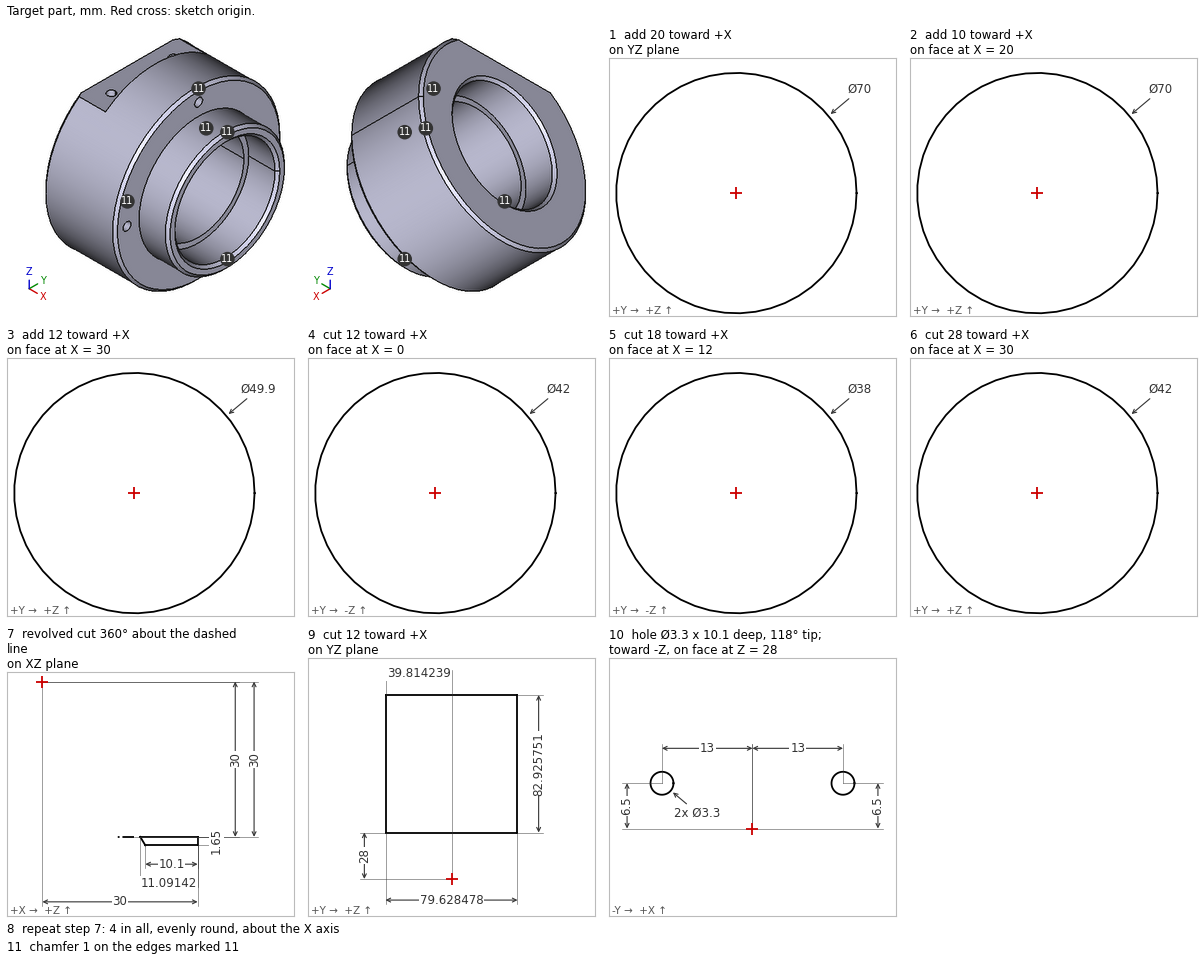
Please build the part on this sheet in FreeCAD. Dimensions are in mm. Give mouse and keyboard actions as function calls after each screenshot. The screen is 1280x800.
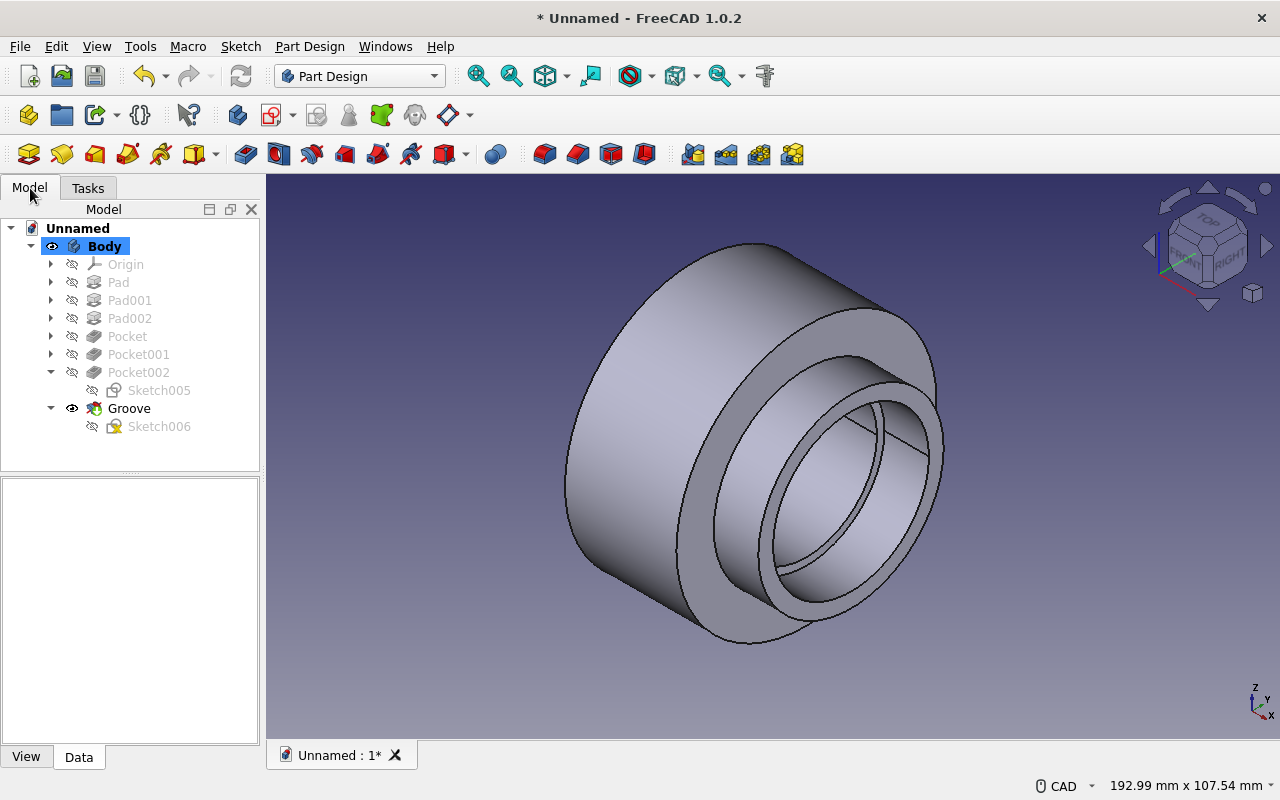
click(117, 408)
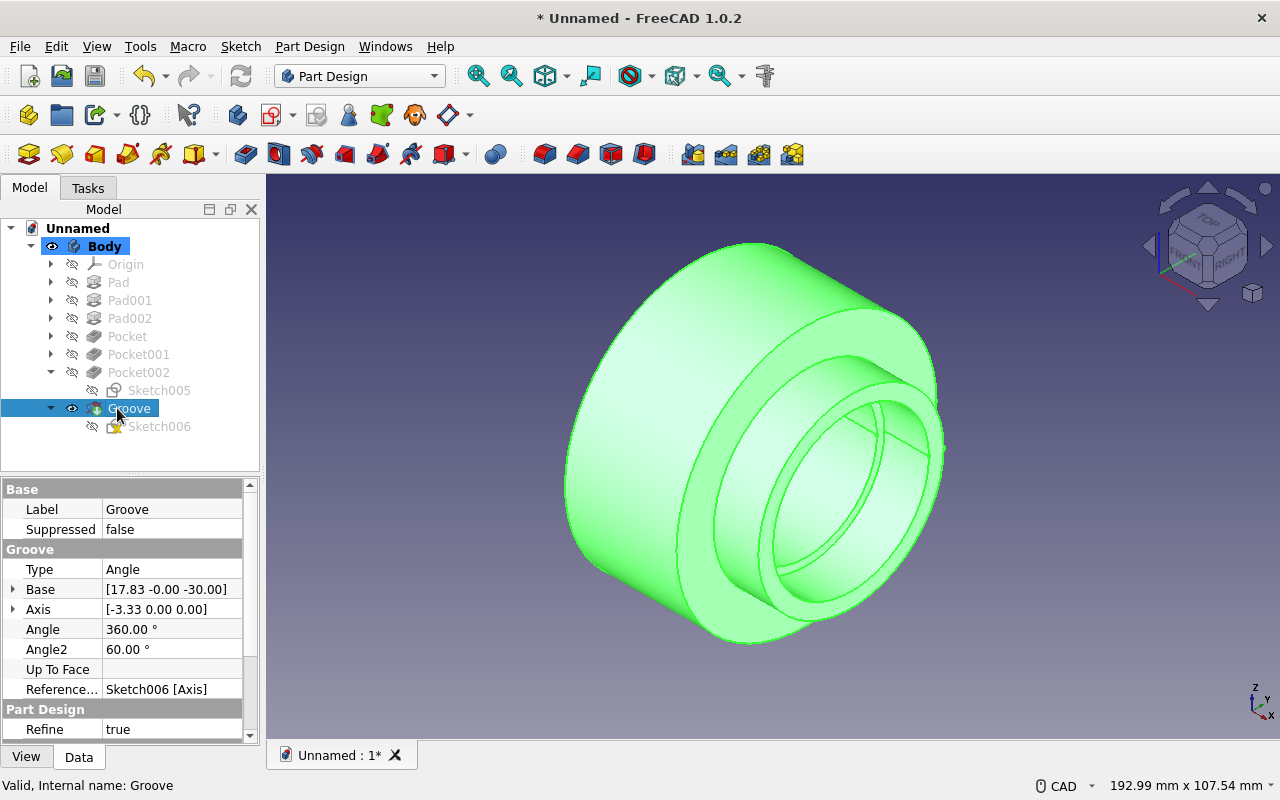
click(759, 154)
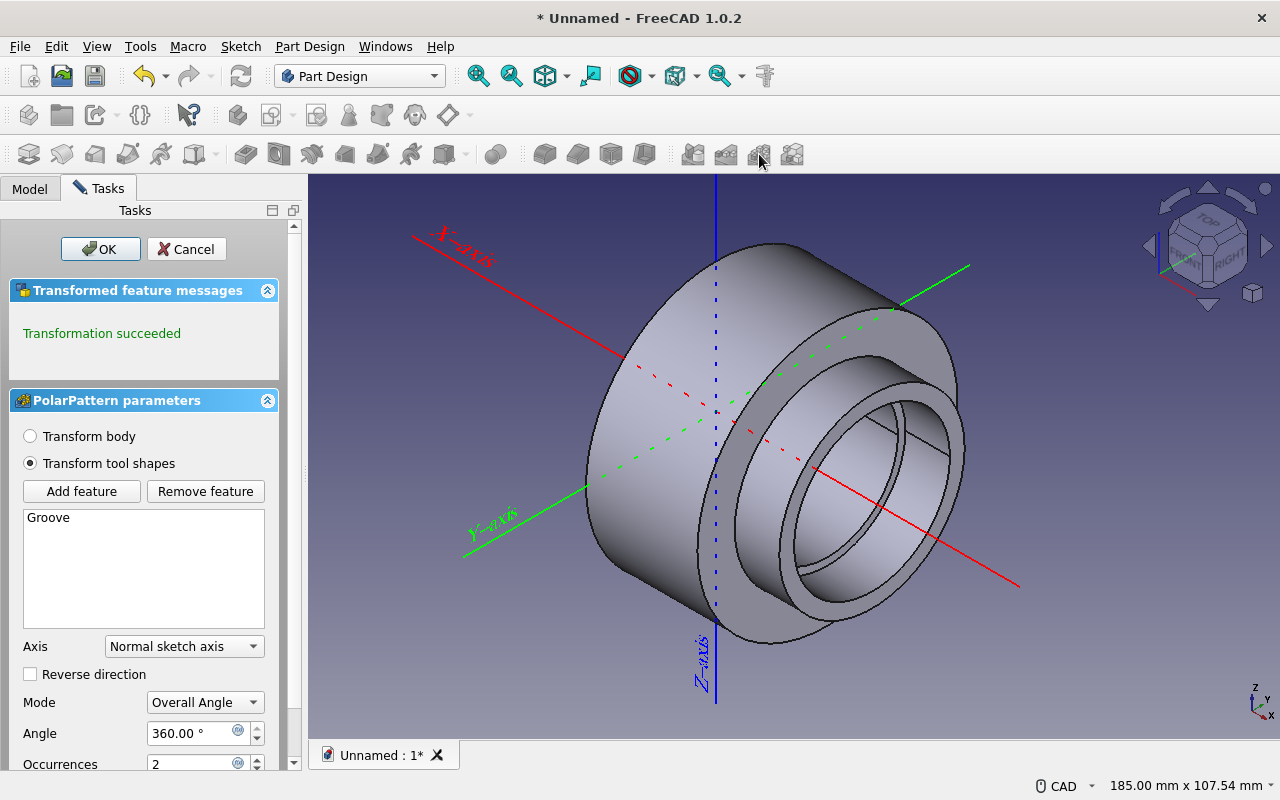
click(185, 646)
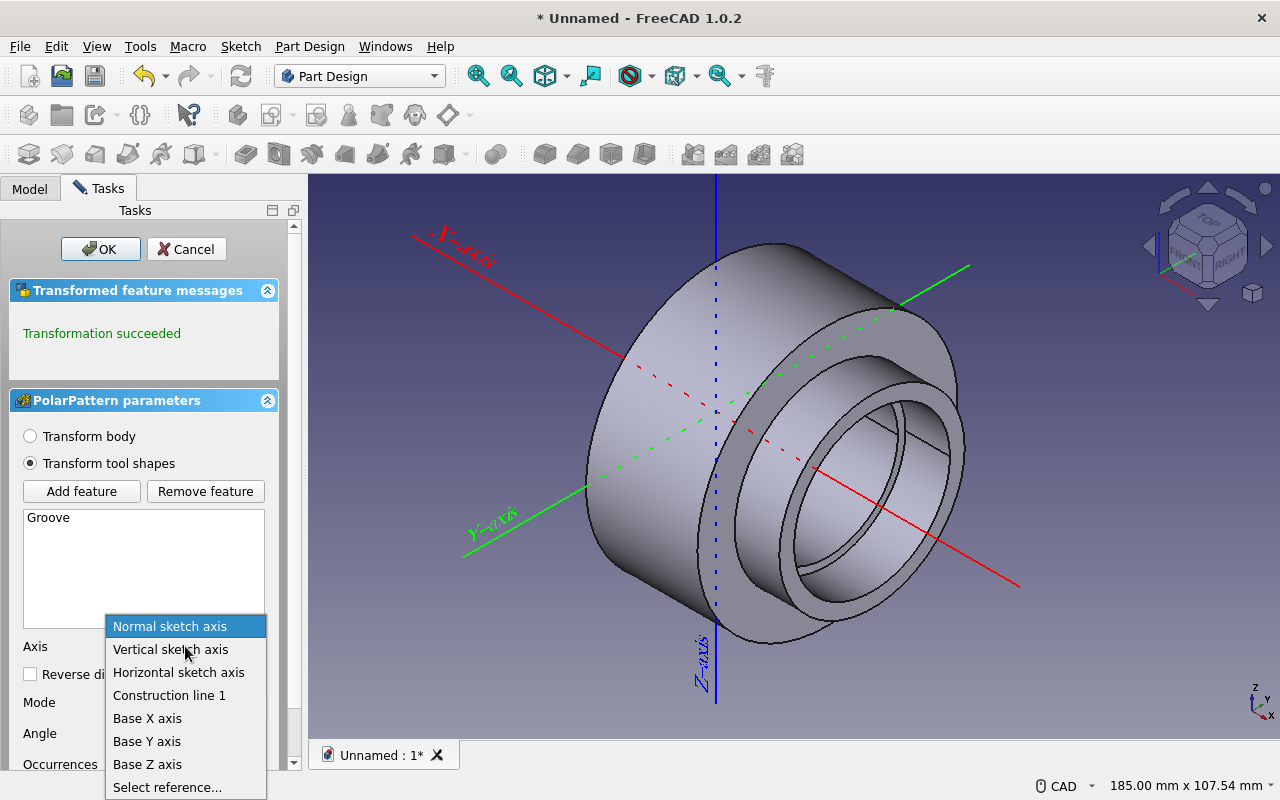
click(184, 718)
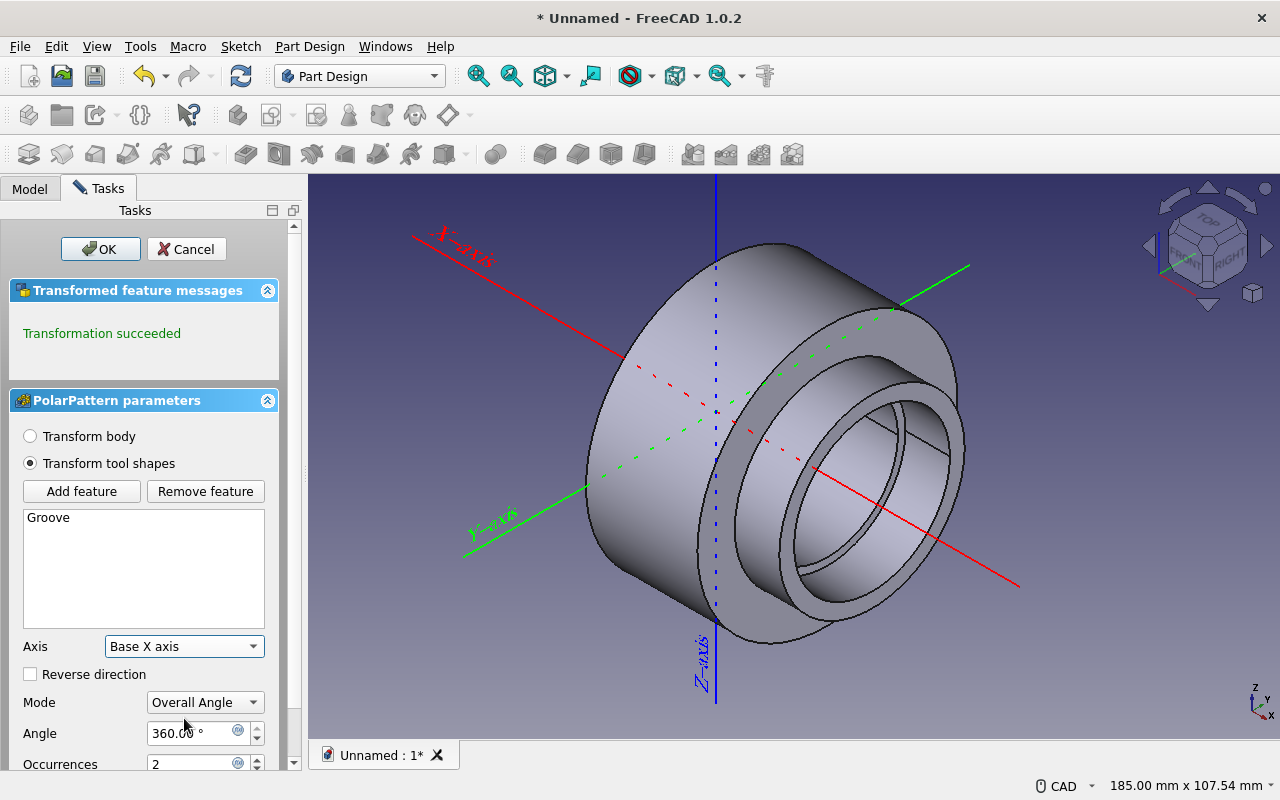
scroll(294, 495, down, 2)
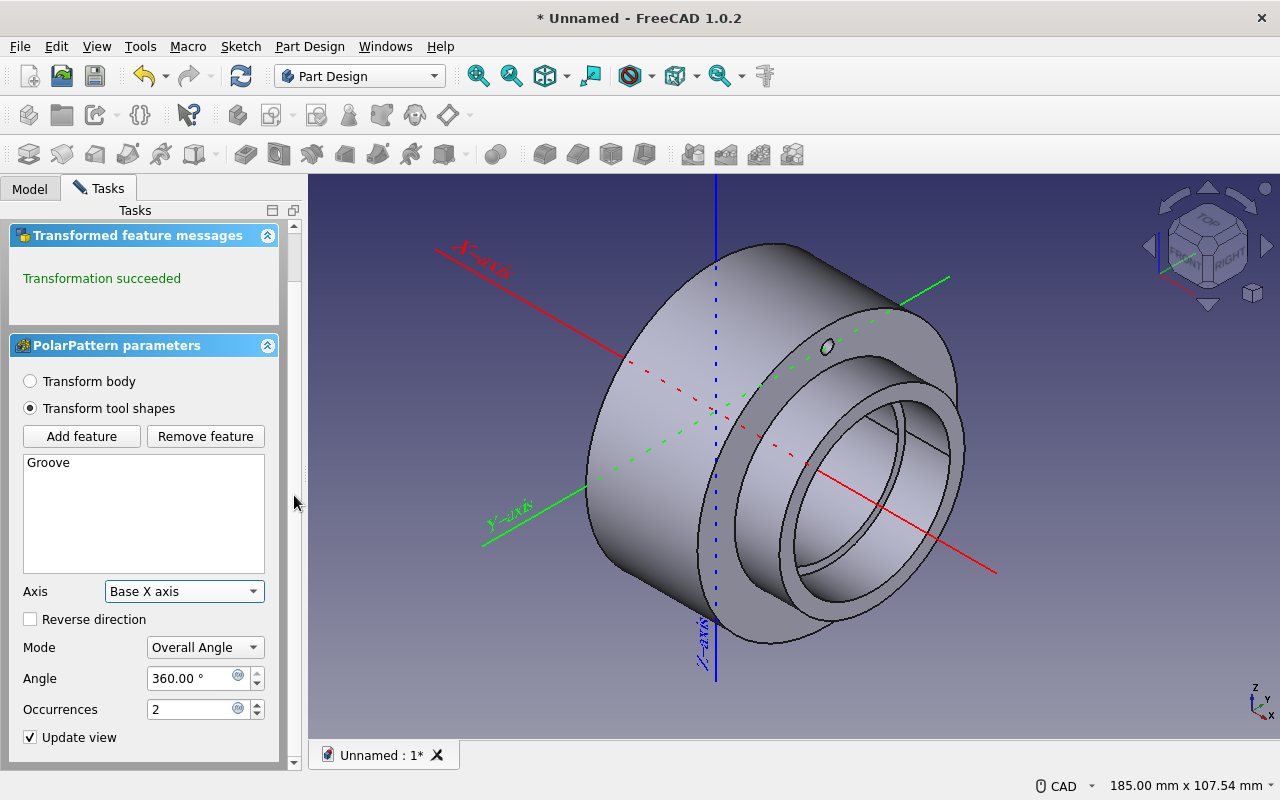
triple_click(199, 710)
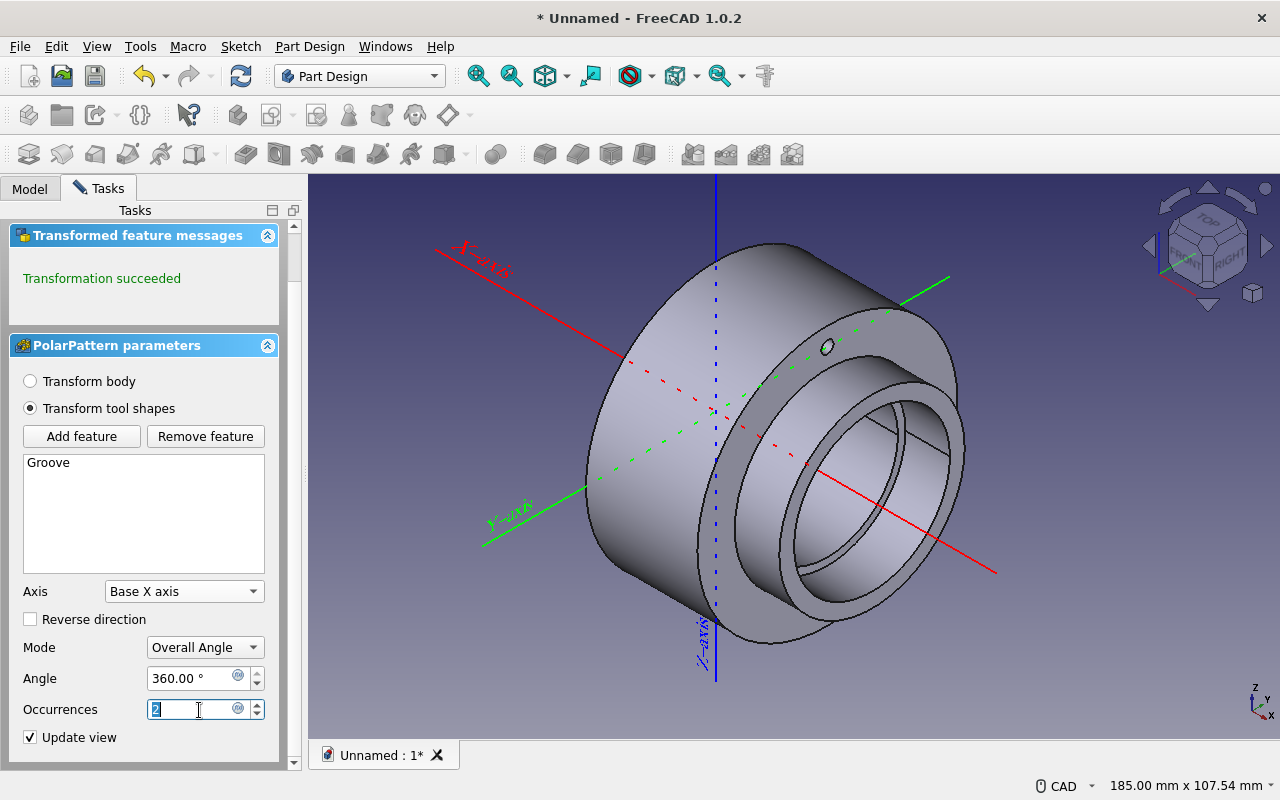
text(4)
key(Tab)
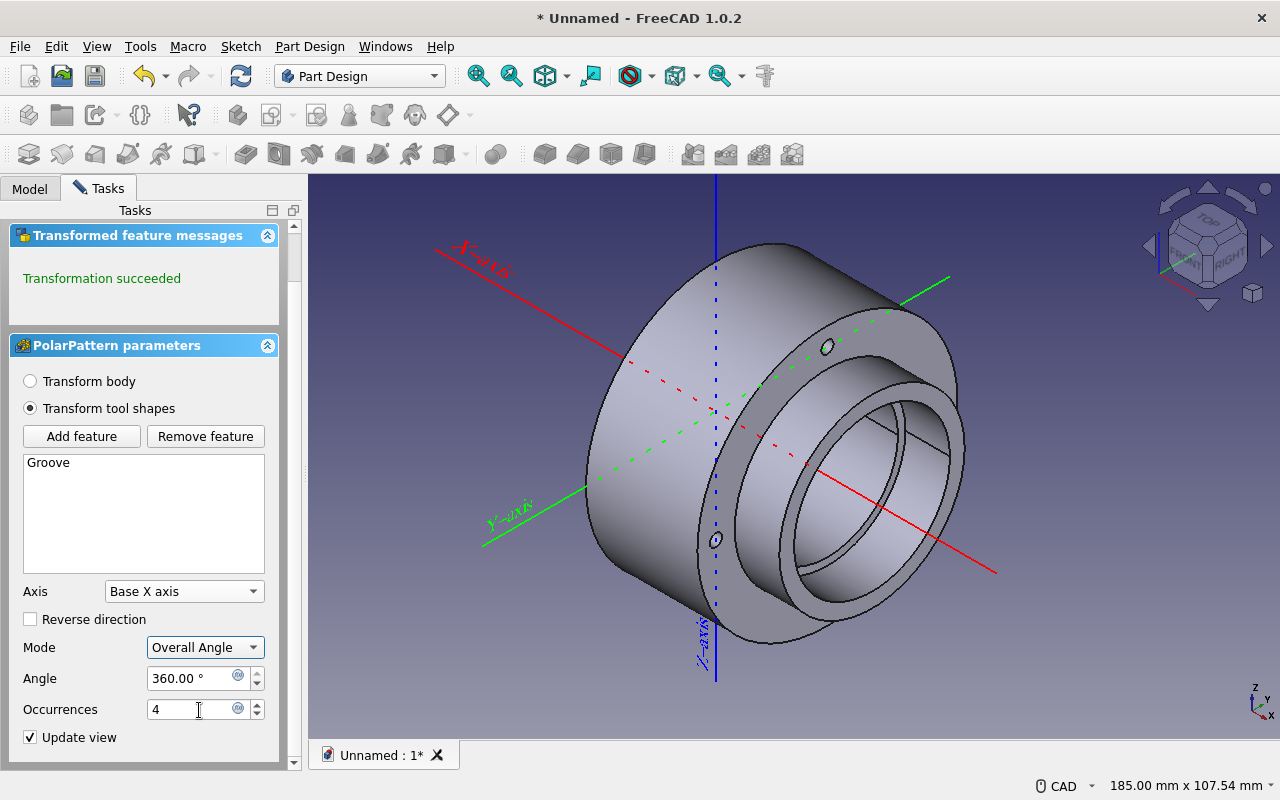
scroll(294, 495, up, 2)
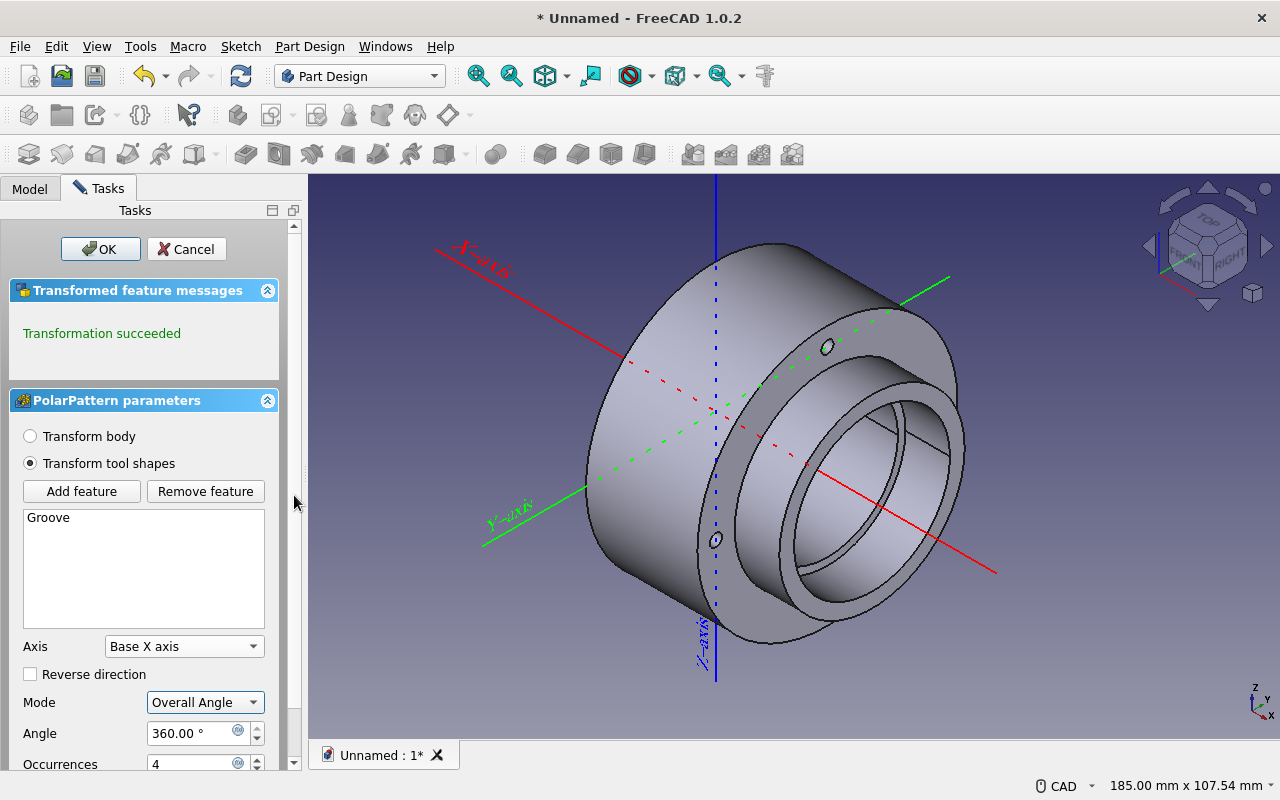
click(101, 249)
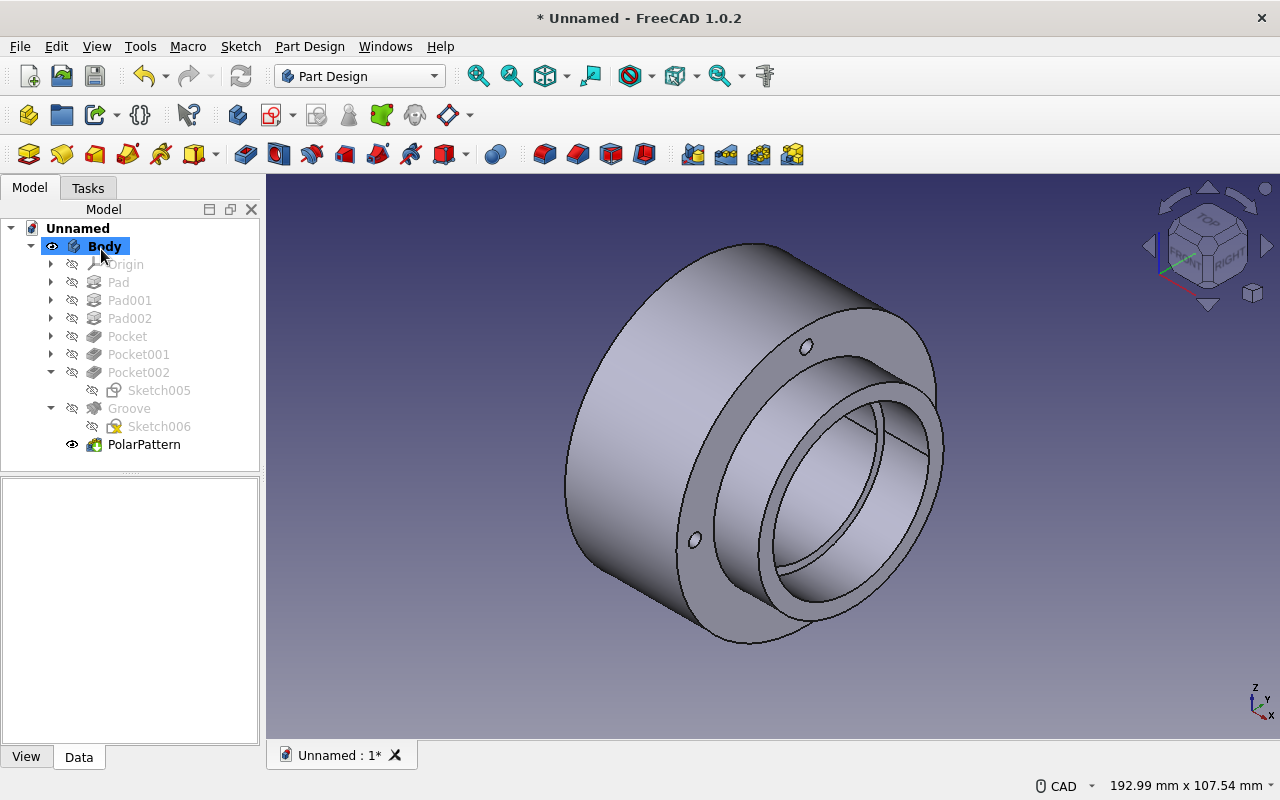
click(270, 116)